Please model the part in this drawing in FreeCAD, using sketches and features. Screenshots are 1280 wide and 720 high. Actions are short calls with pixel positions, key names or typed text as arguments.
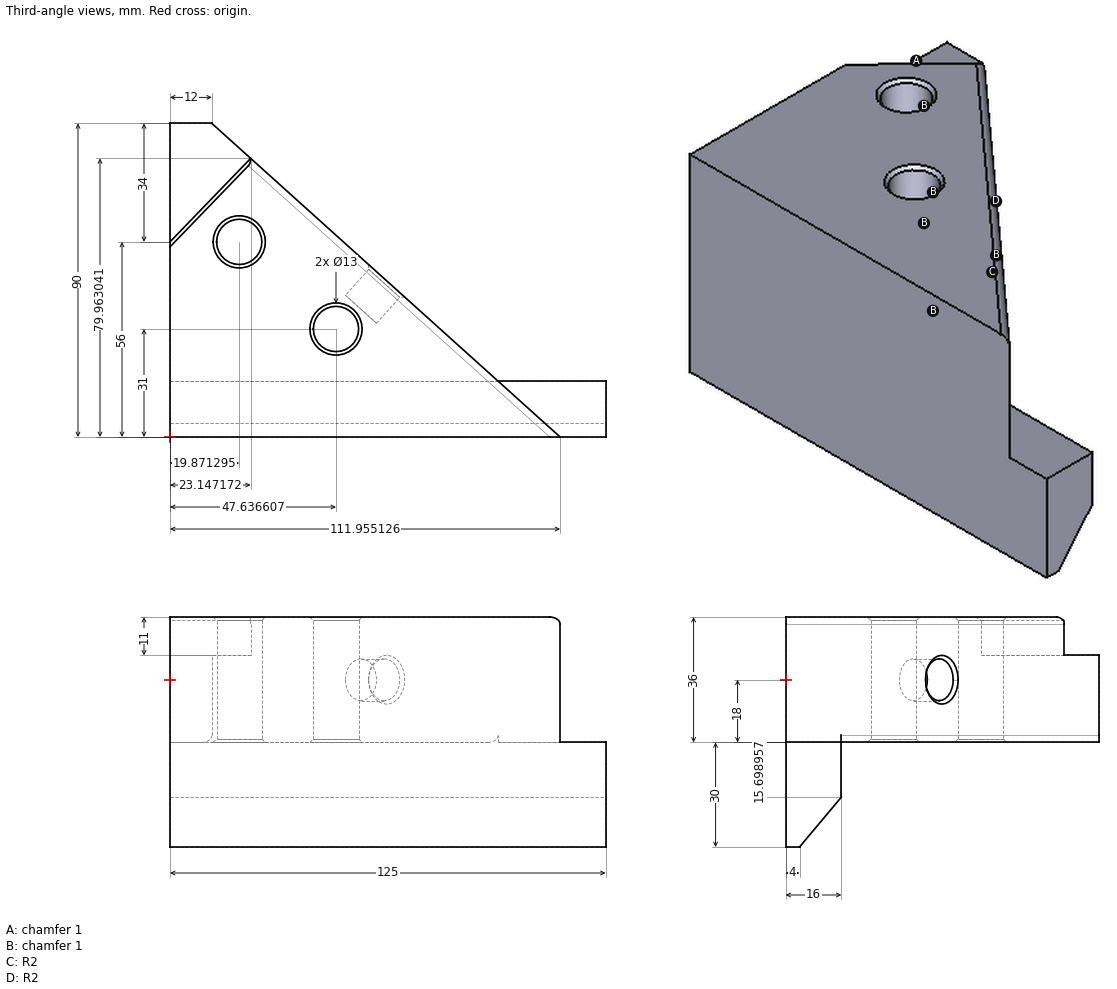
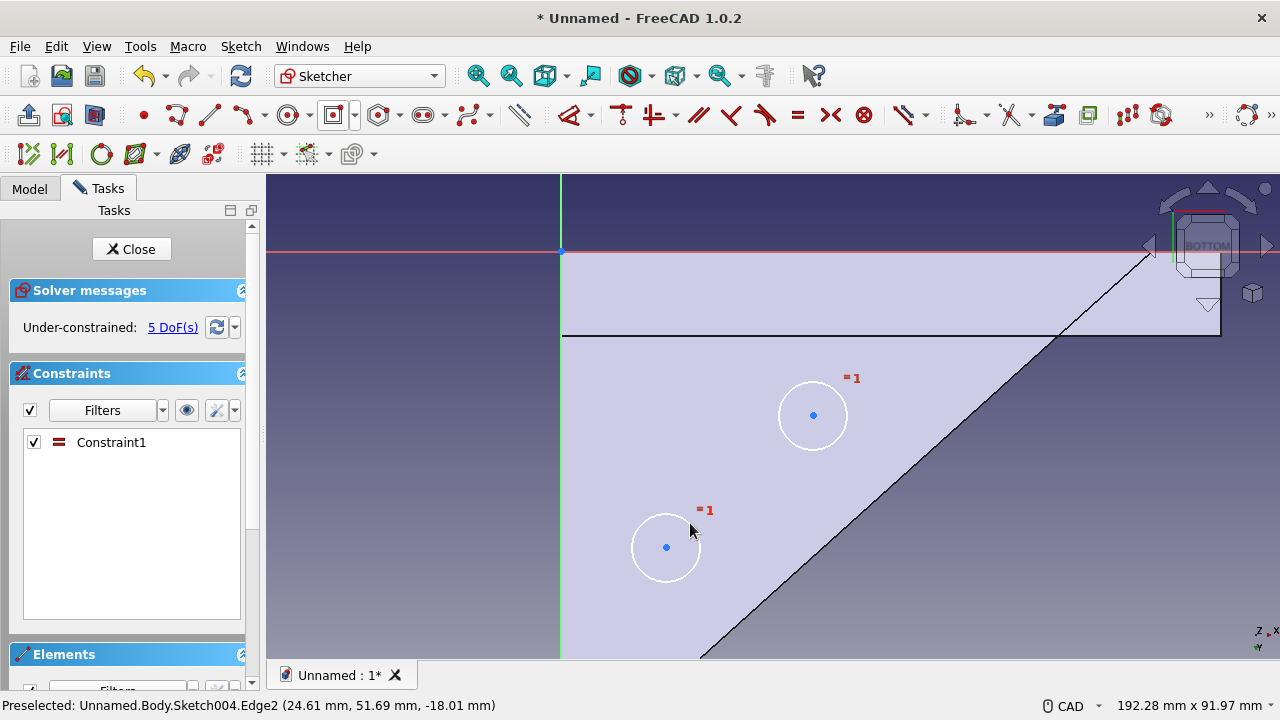
click(568, 116)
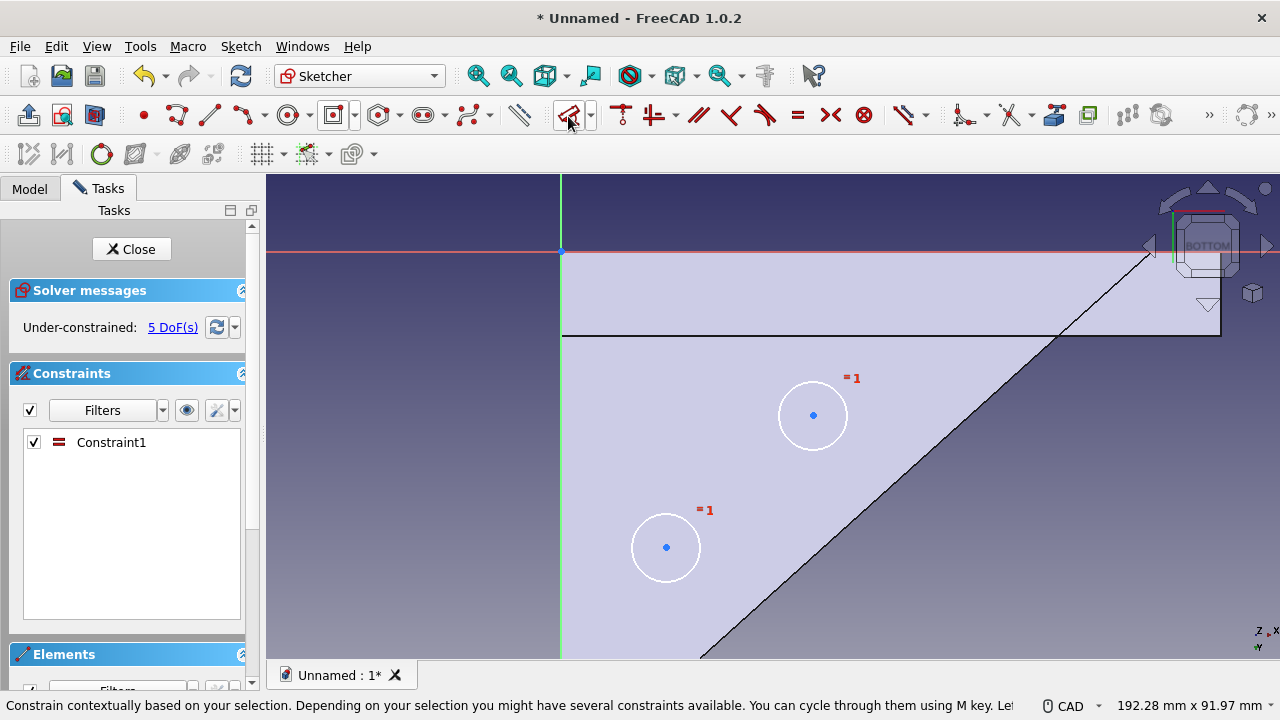
click(837, 392)
click(860, 369)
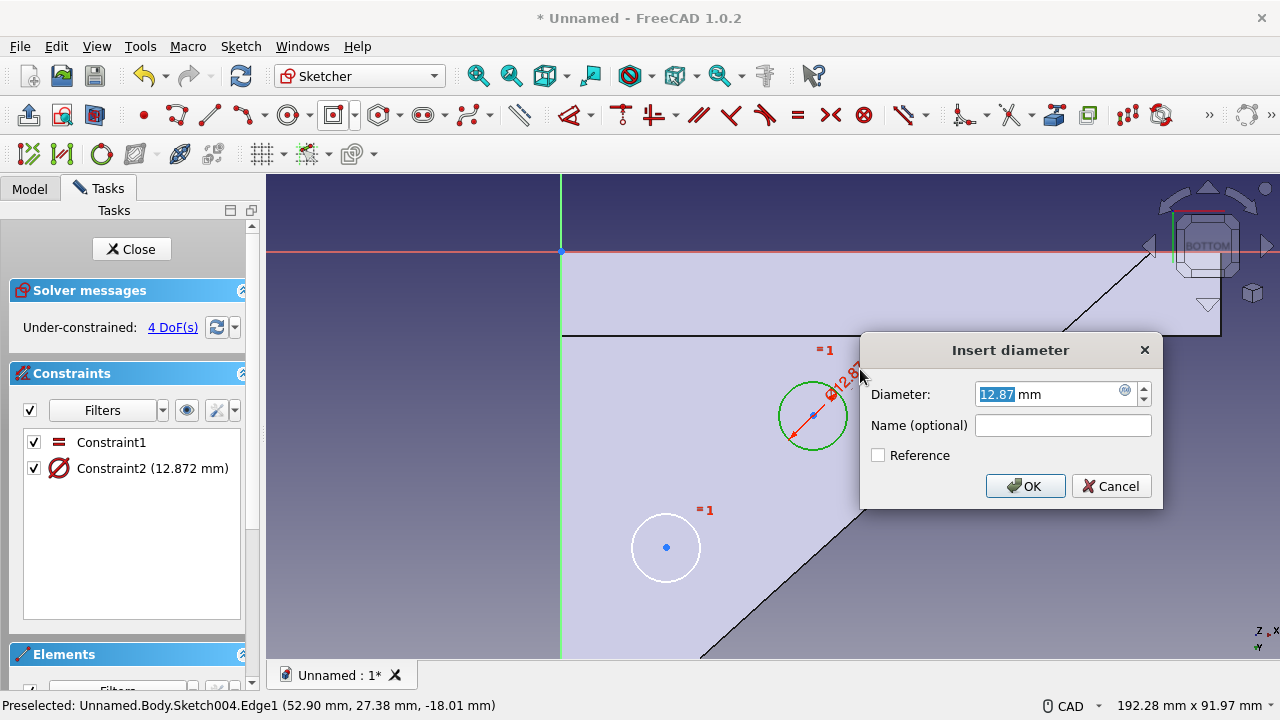
text(13)
key(Return)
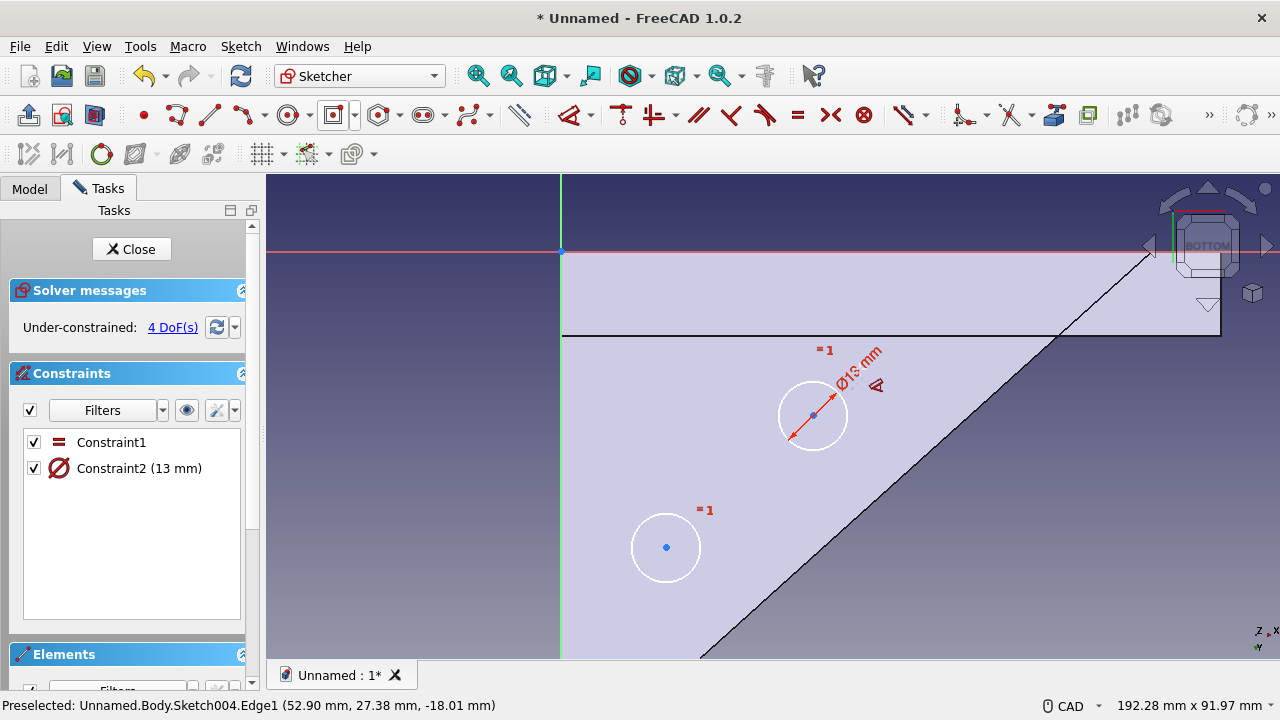
click(813, 416)
click(527, 334)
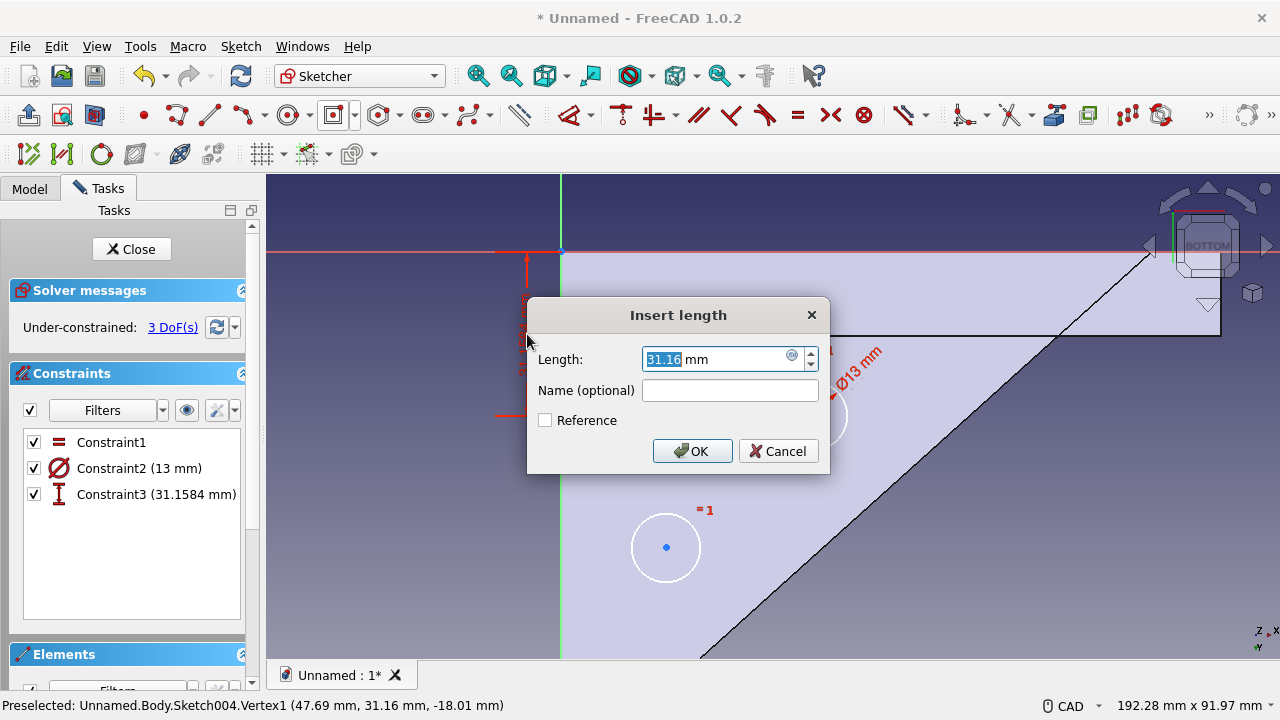
text(31)
key(Return)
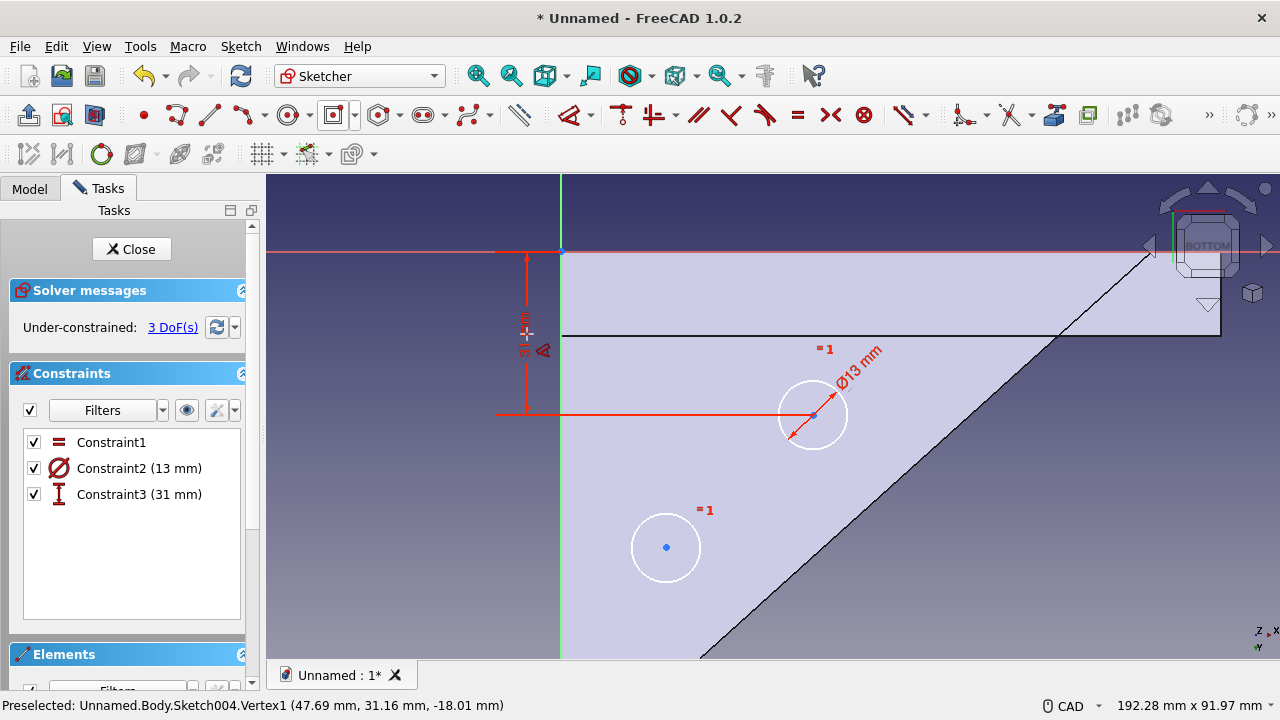
click(666, 548)
click(527, 400)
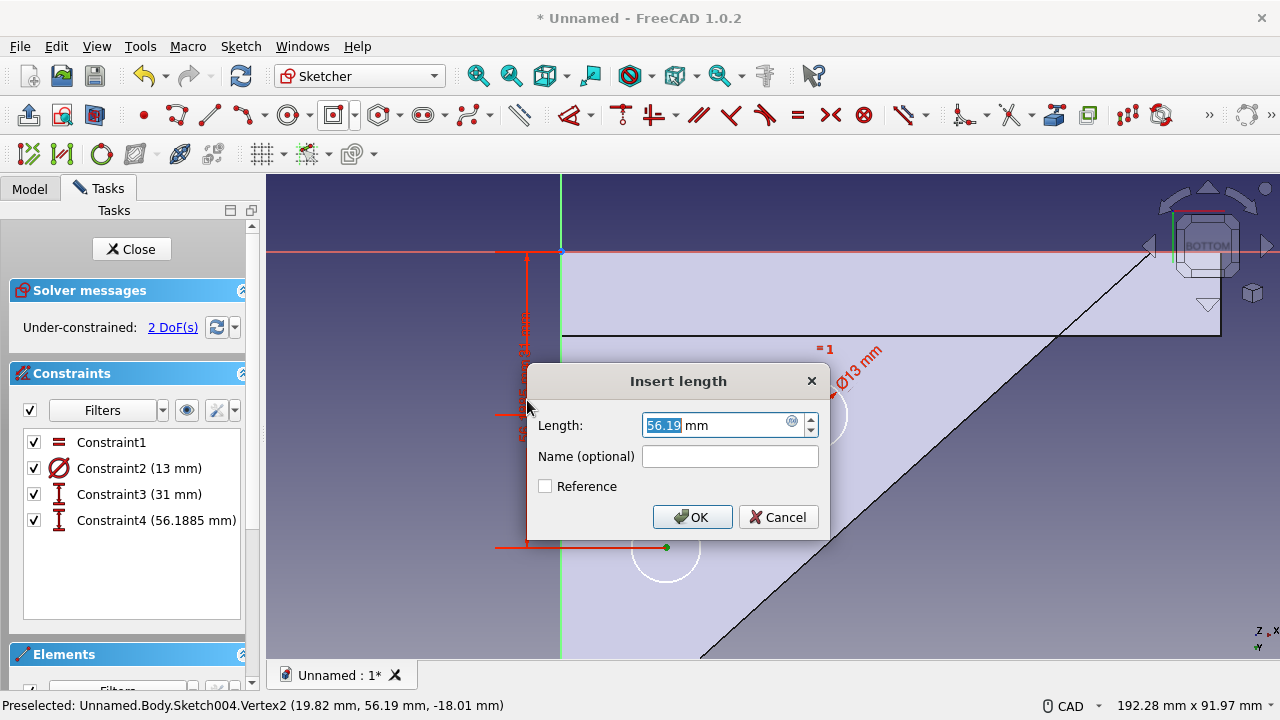
text(56)
key(Return)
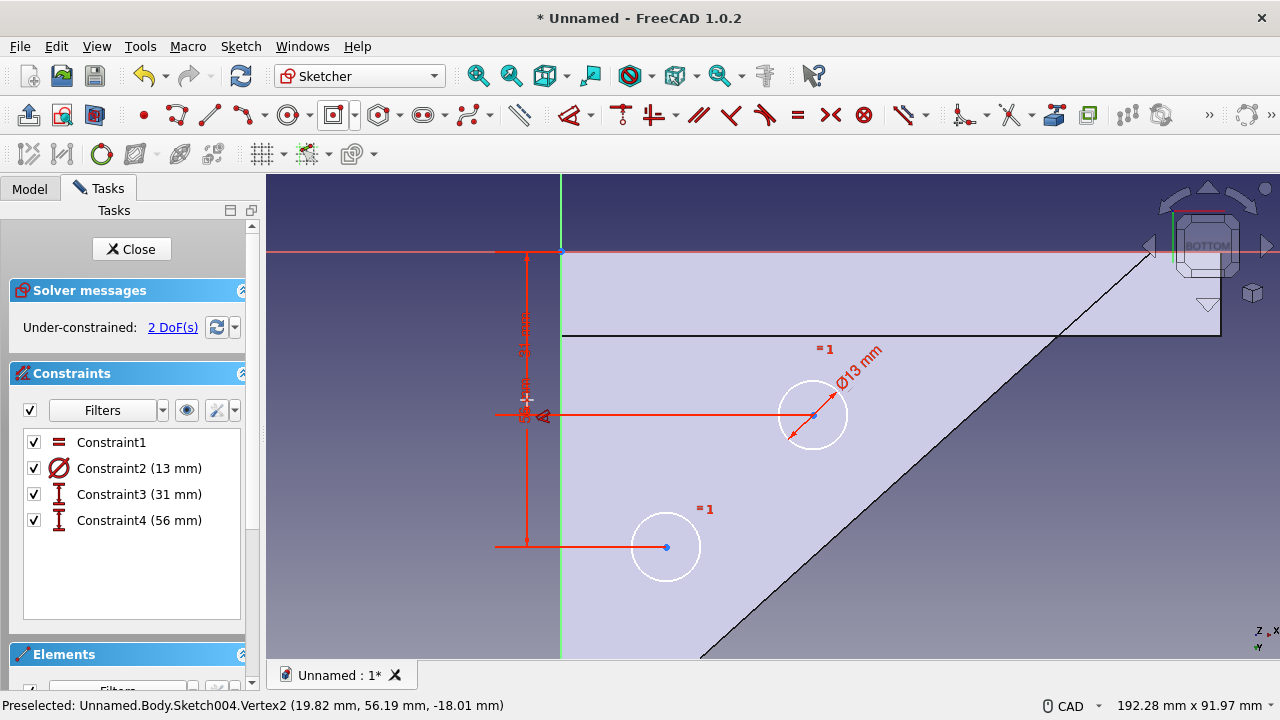
click(813, 415)
click(687, 218)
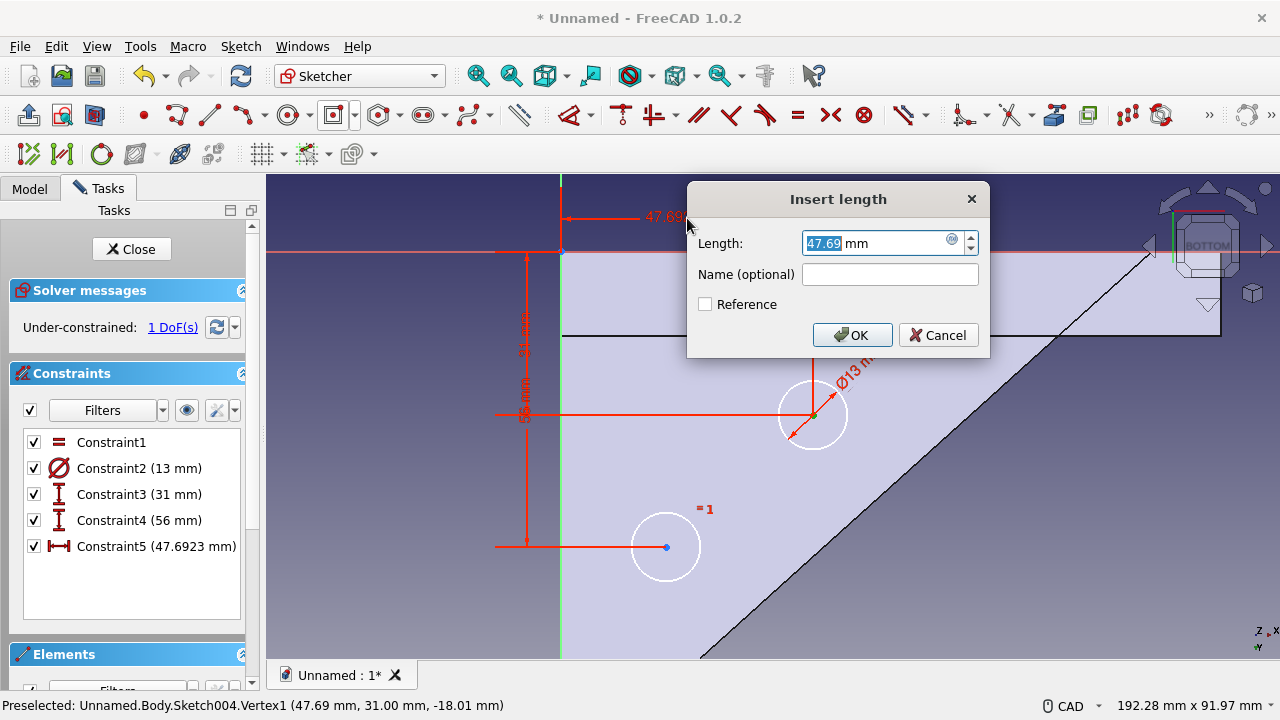
text(47.636607)
key(Return)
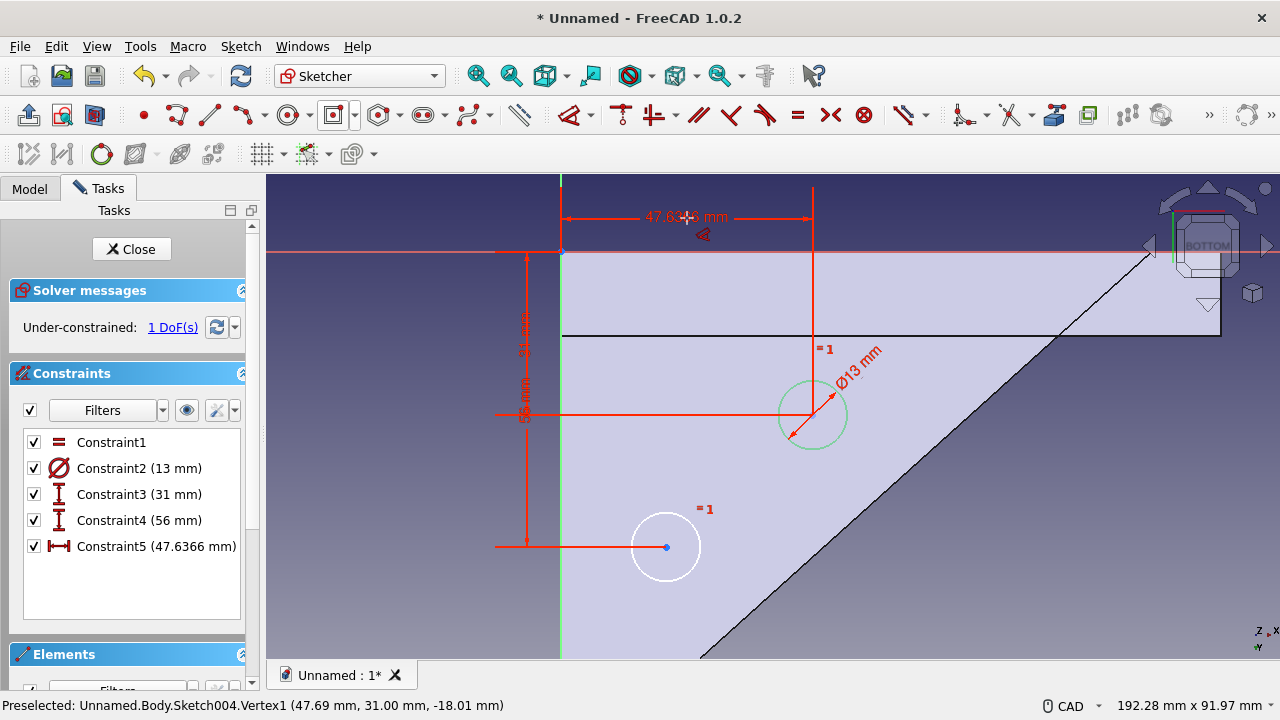
click(666, 547)
click(614, 218)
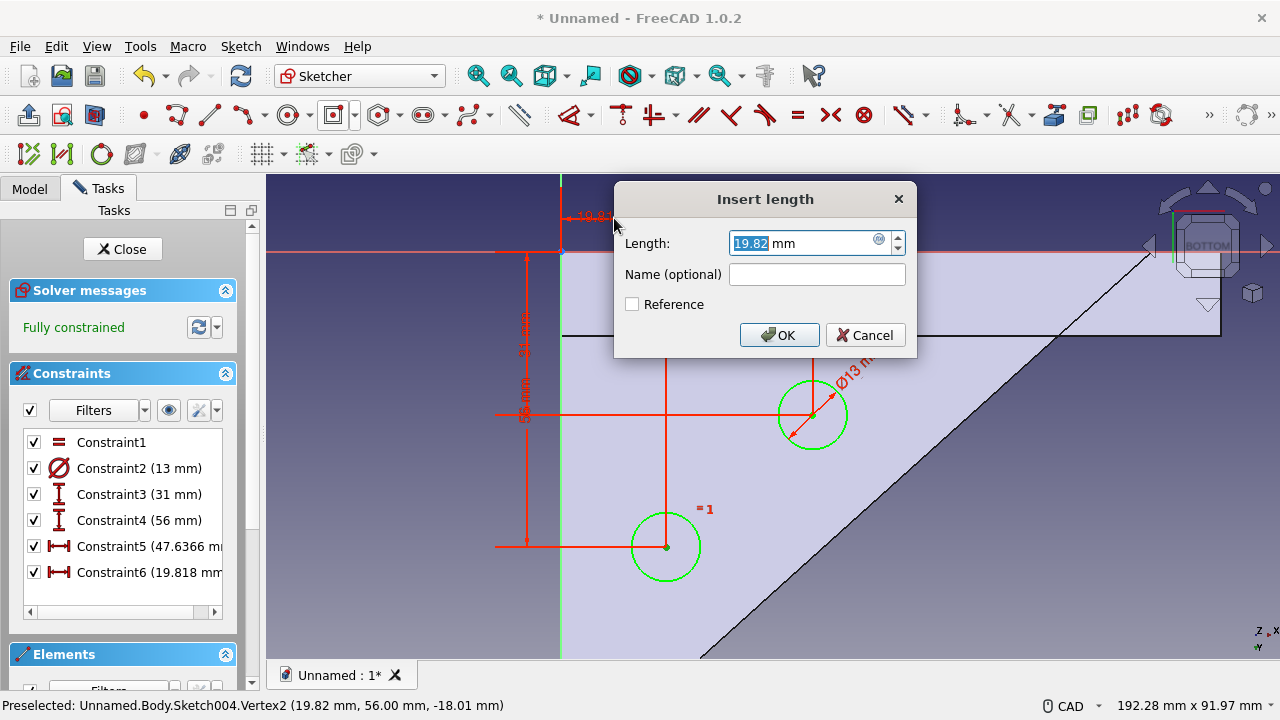
text(19.871295)
key(Return)
key(Escape)